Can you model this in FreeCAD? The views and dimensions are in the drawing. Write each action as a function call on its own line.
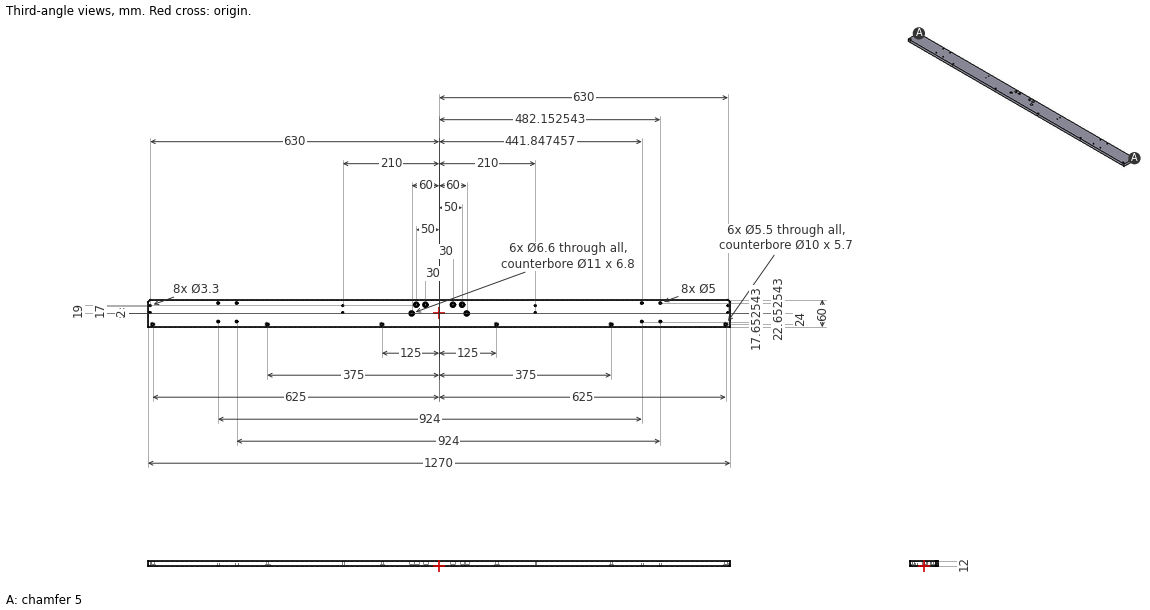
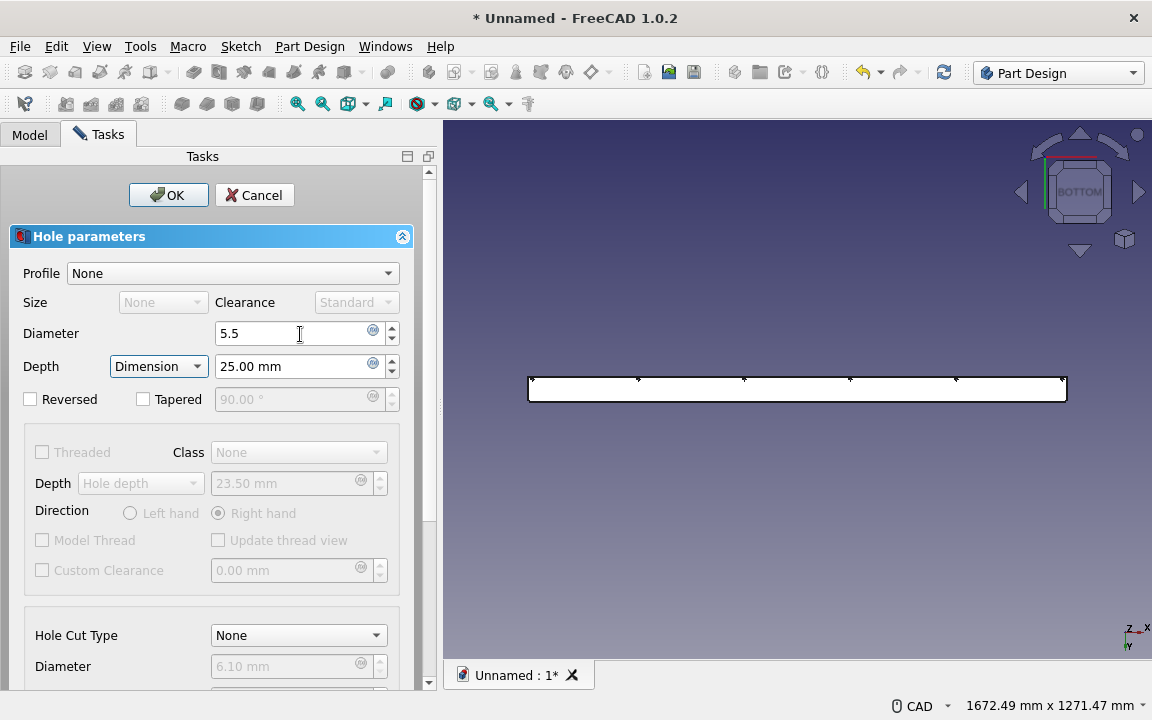
click(160, 366)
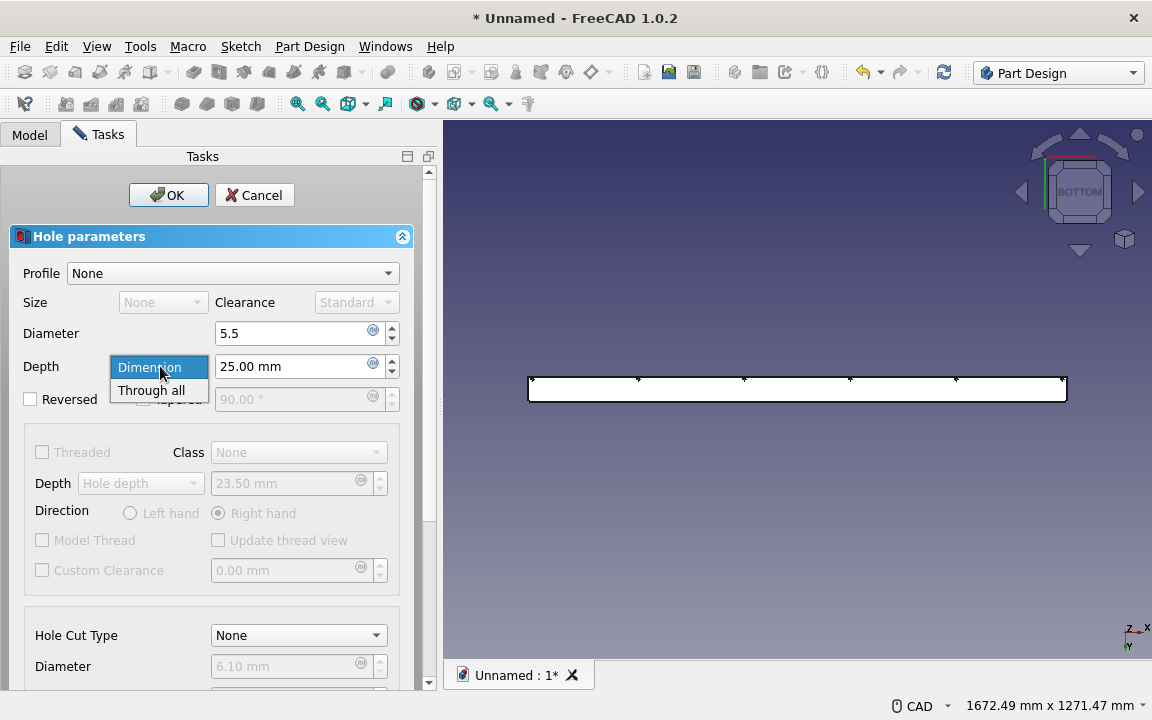
click(158, 390)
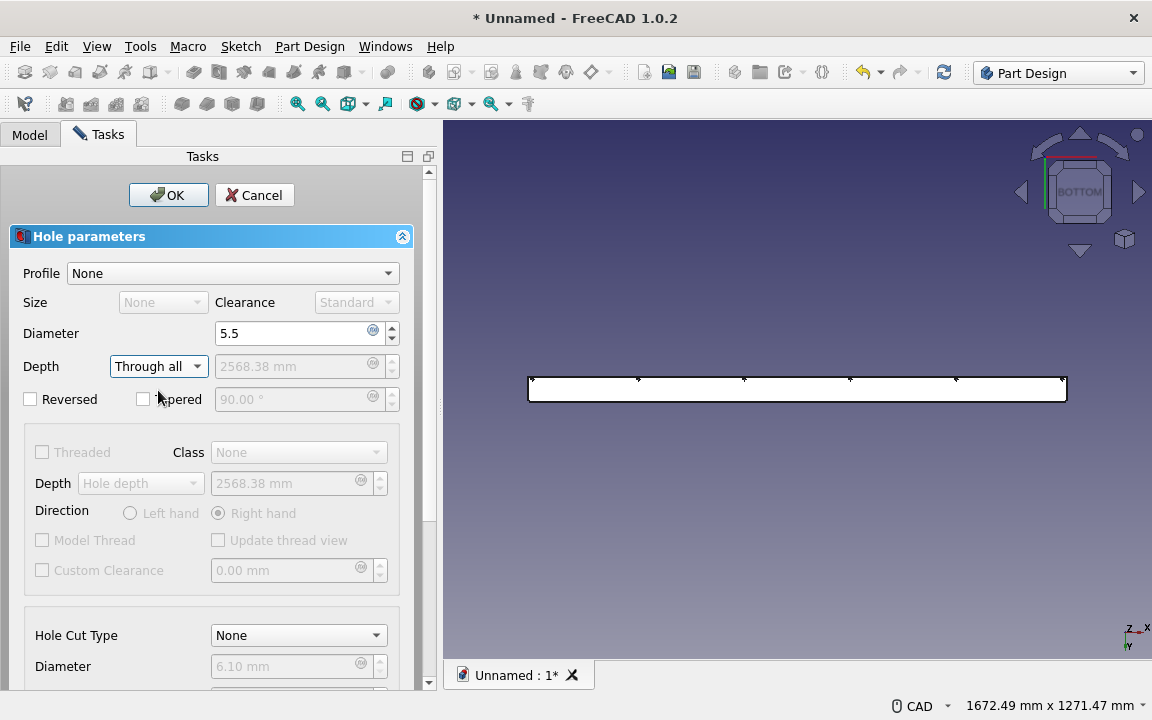
click(300, 636)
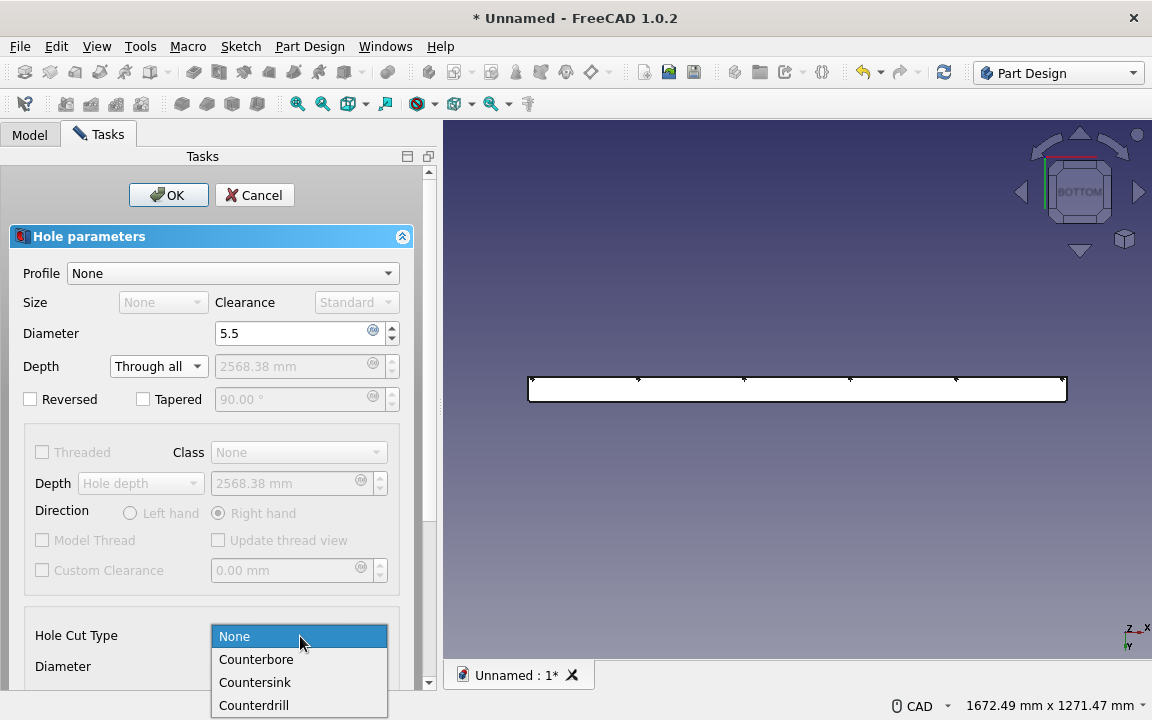
click(298, 660)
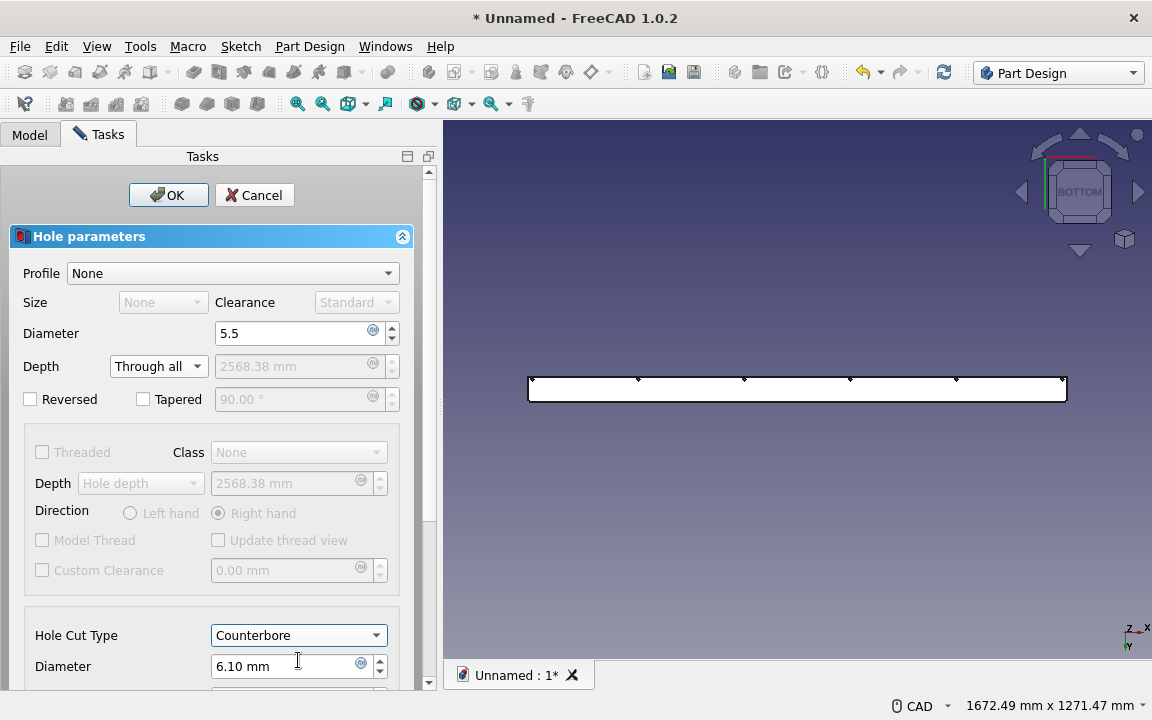
triple_click(292, 666)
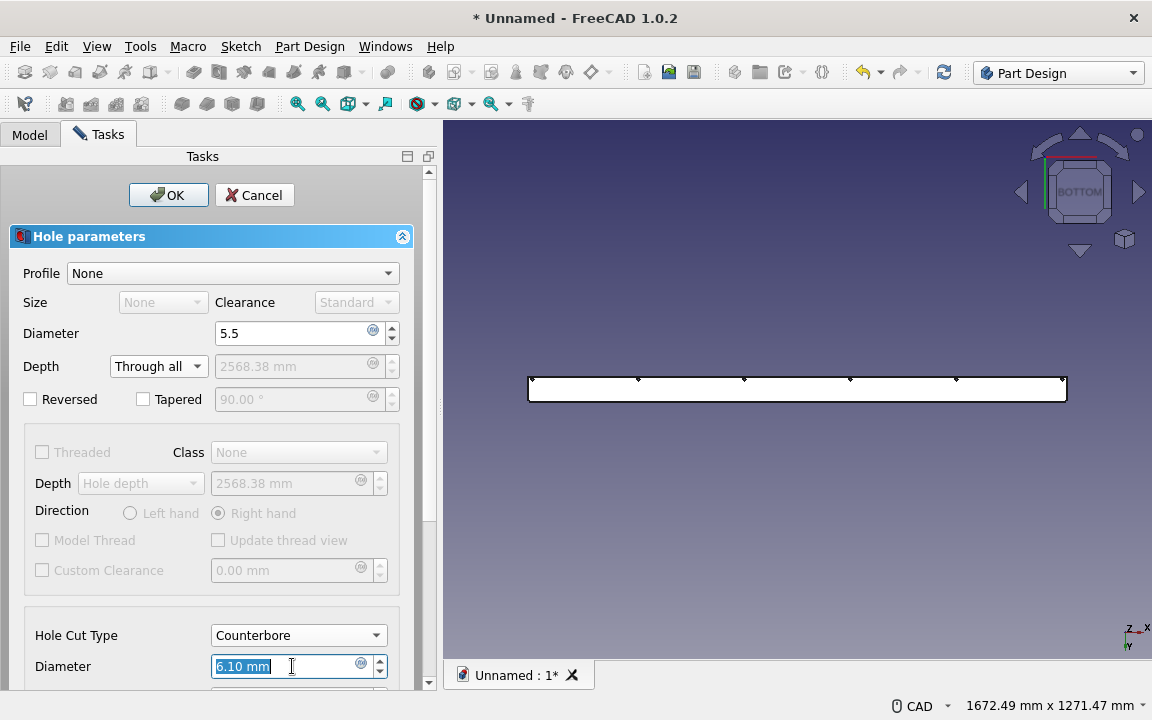
text(10)
key(Tab)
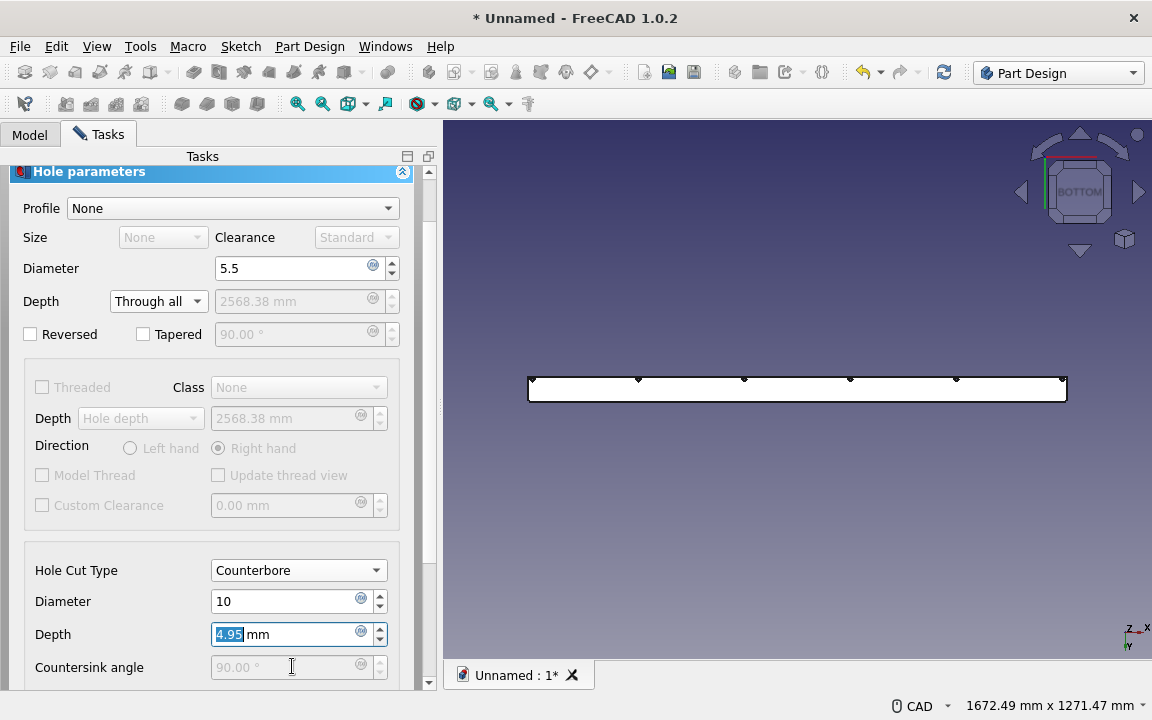
text(5.7)
key(Tab)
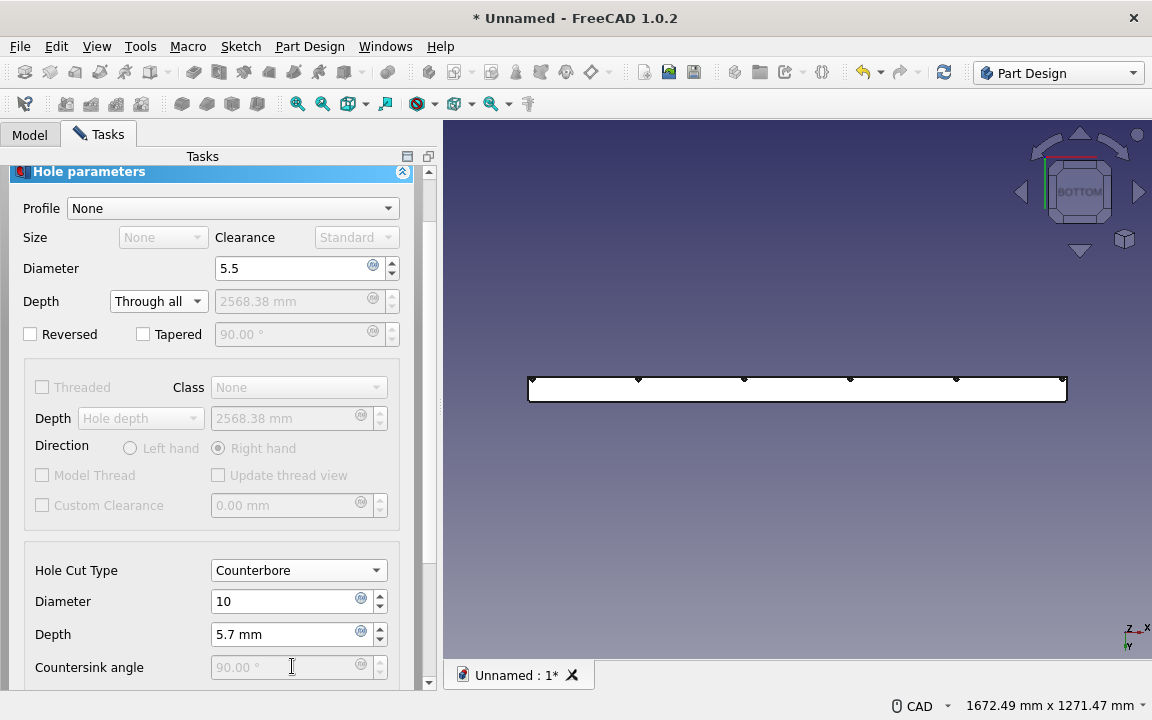
scroll(429, 428, up, 2)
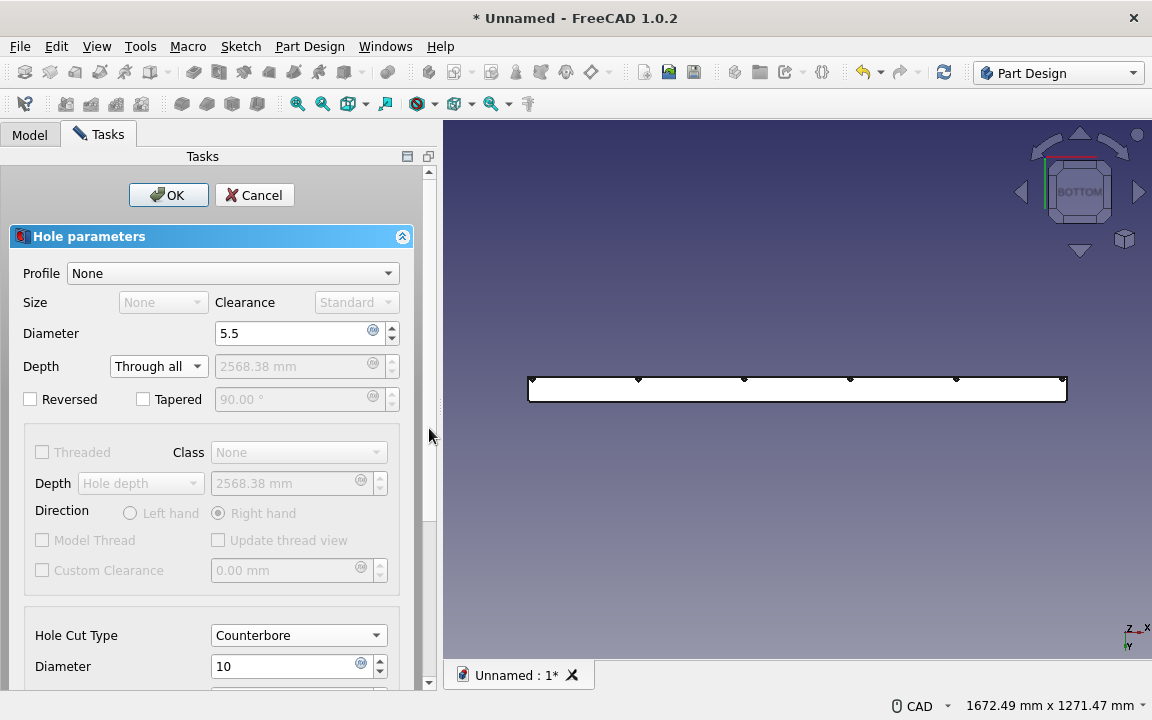
click(169, 195)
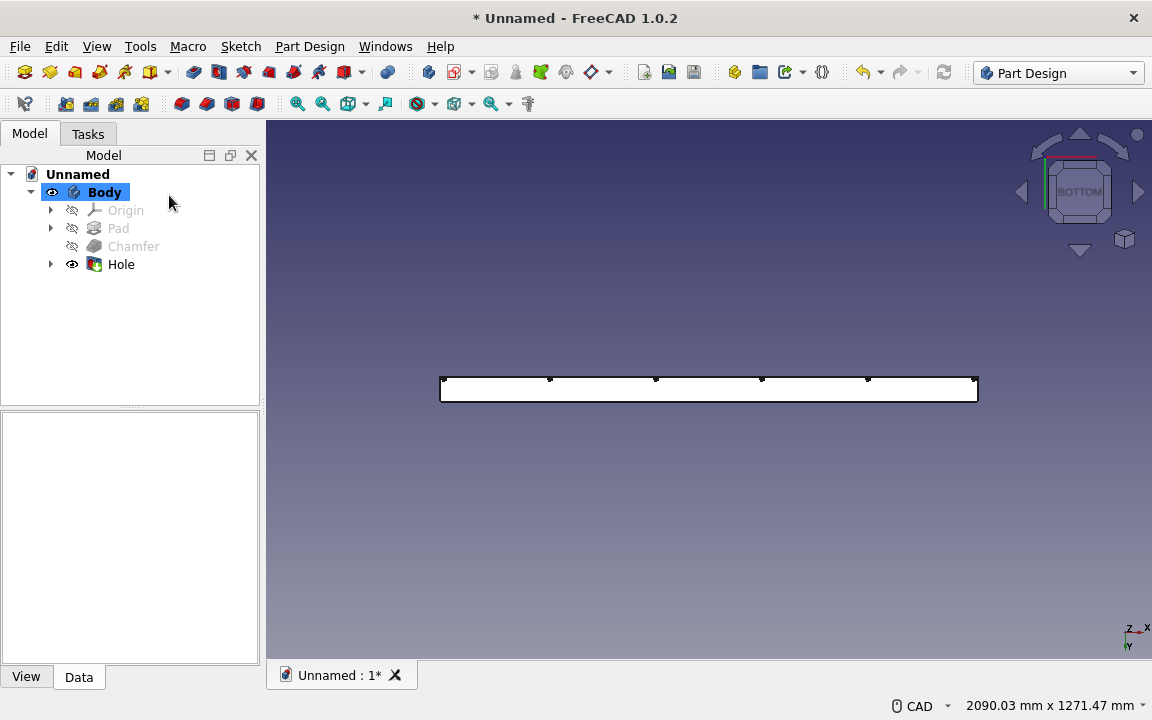
click(940, 389)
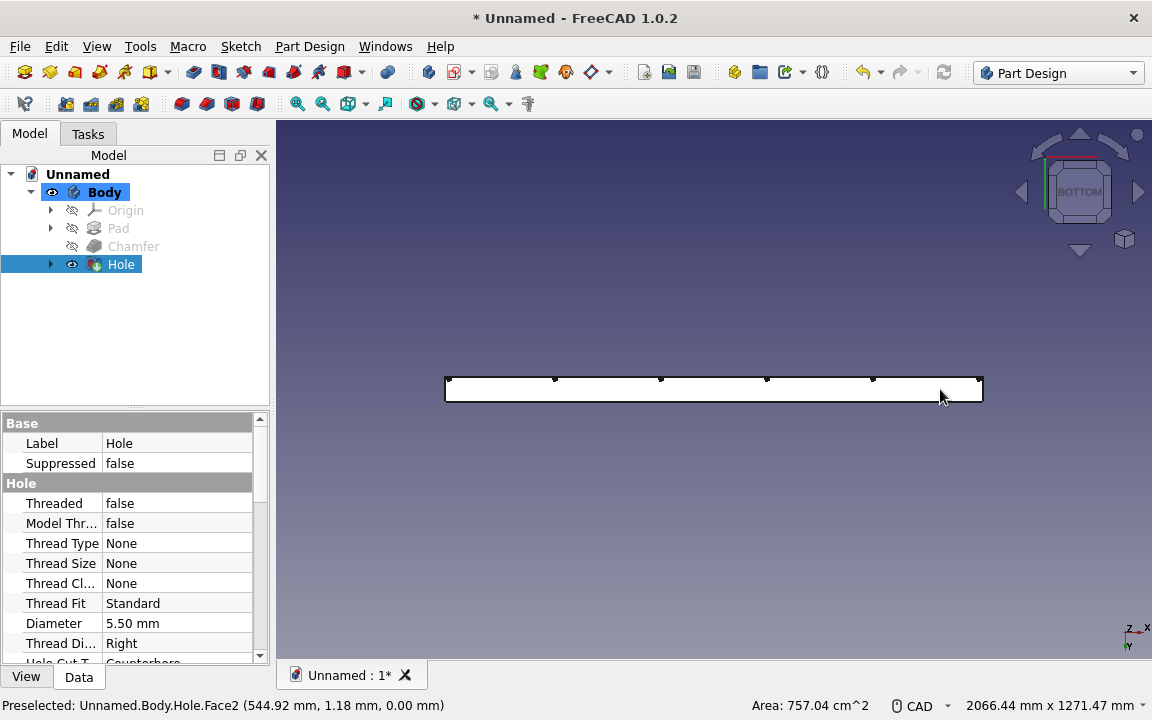
click(454, 72)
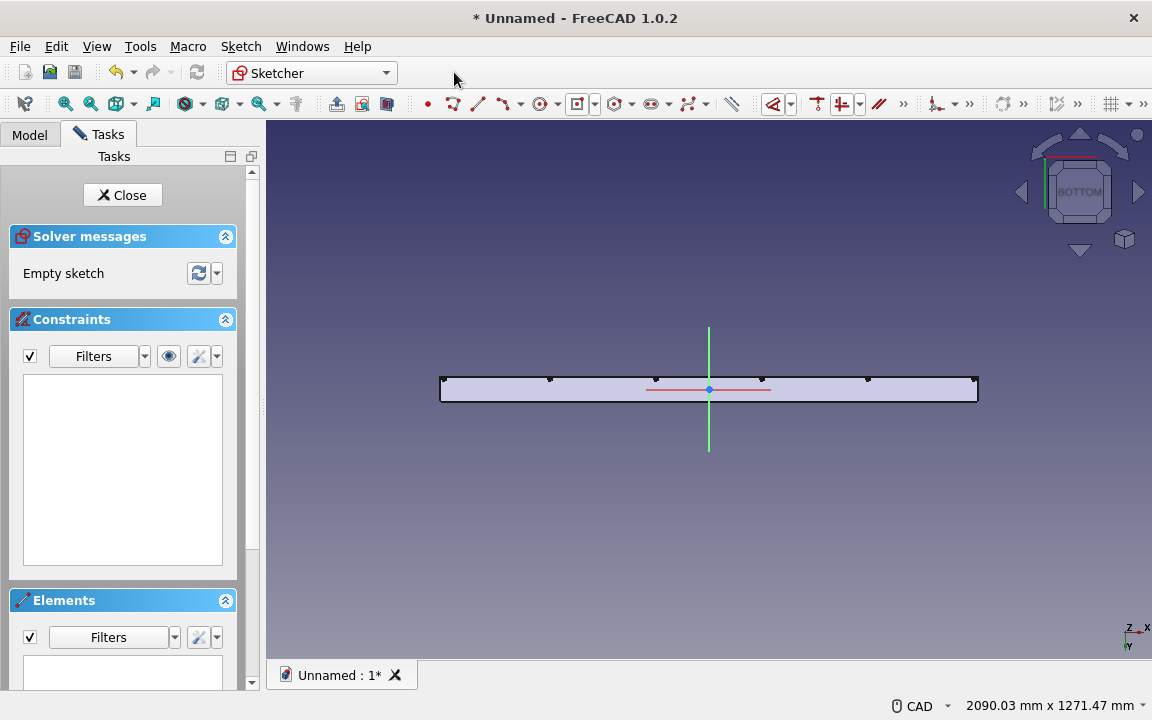
click(540, 104)